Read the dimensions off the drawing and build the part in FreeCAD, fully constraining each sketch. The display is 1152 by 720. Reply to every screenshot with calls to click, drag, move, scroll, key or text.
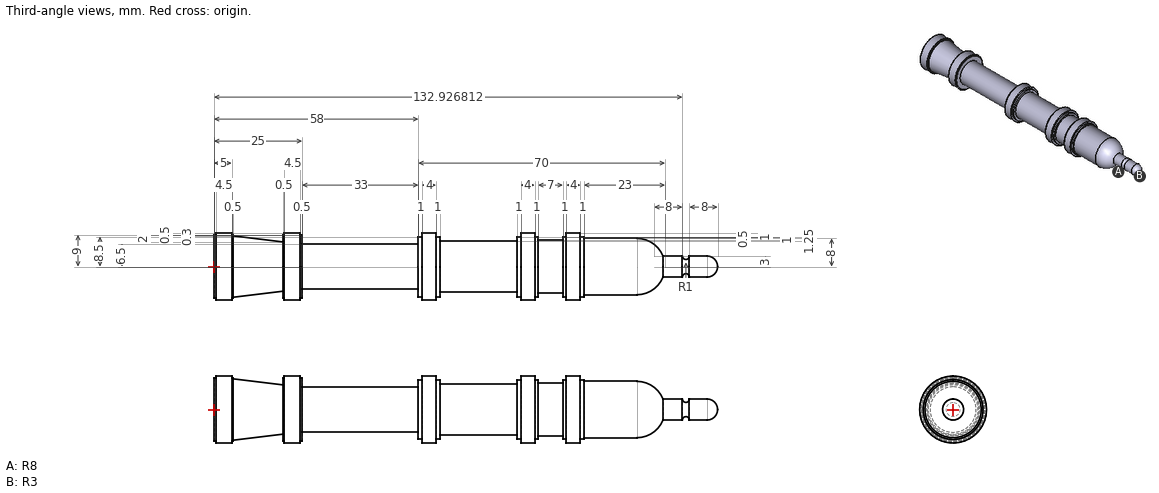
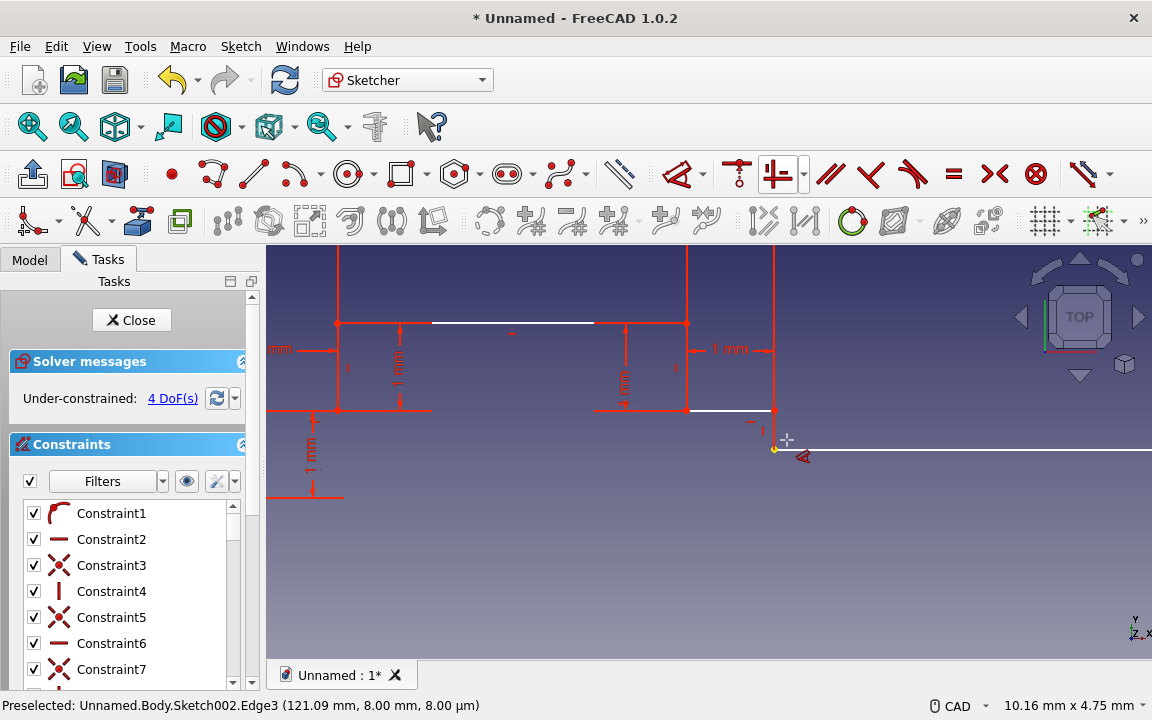
click(774, 430)
click(808, 430)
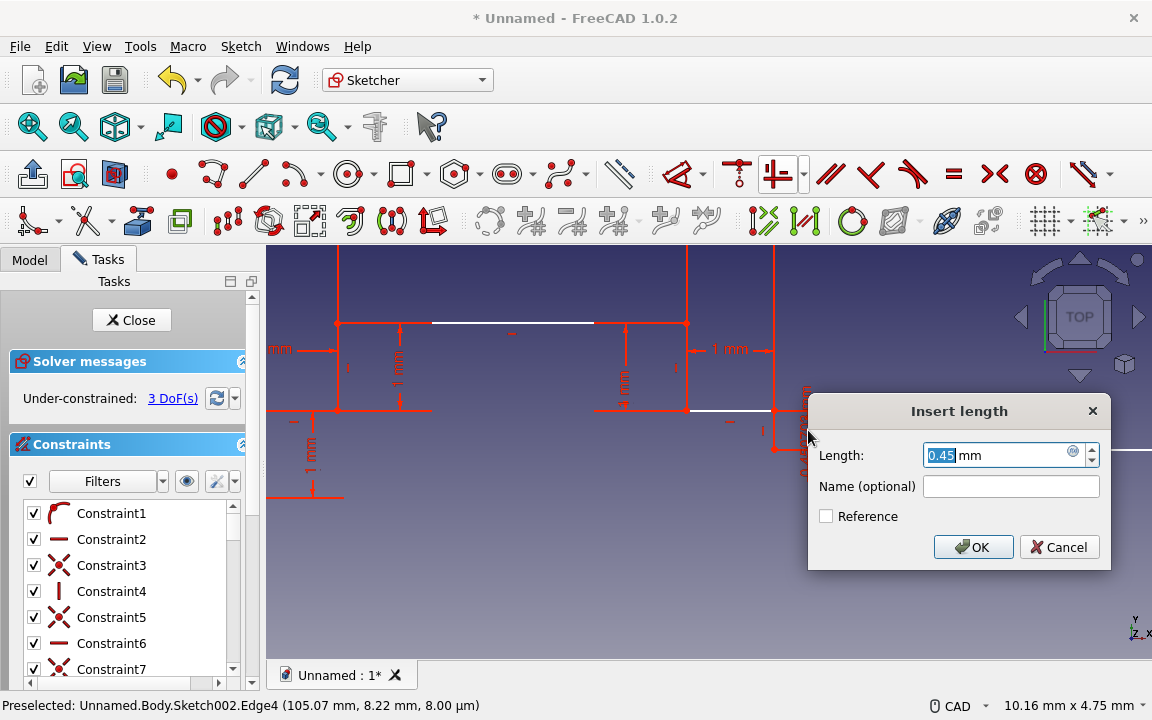
text(0.5)
key(Return)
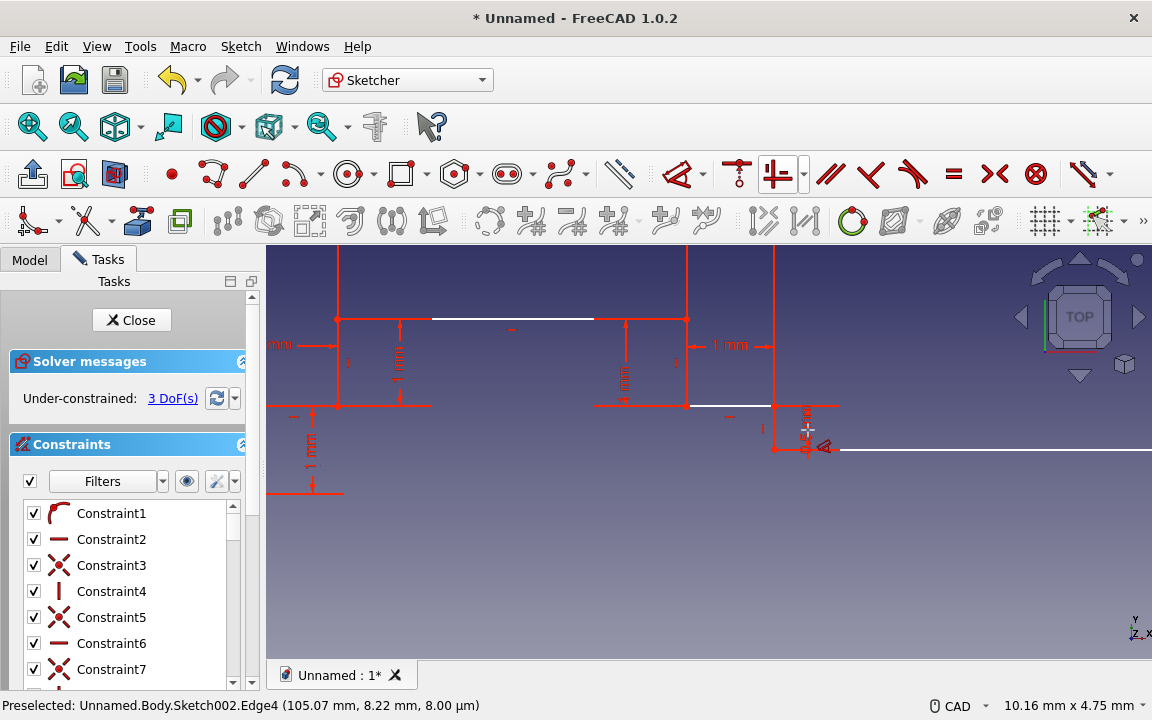
scroll(821, 437, down, 15)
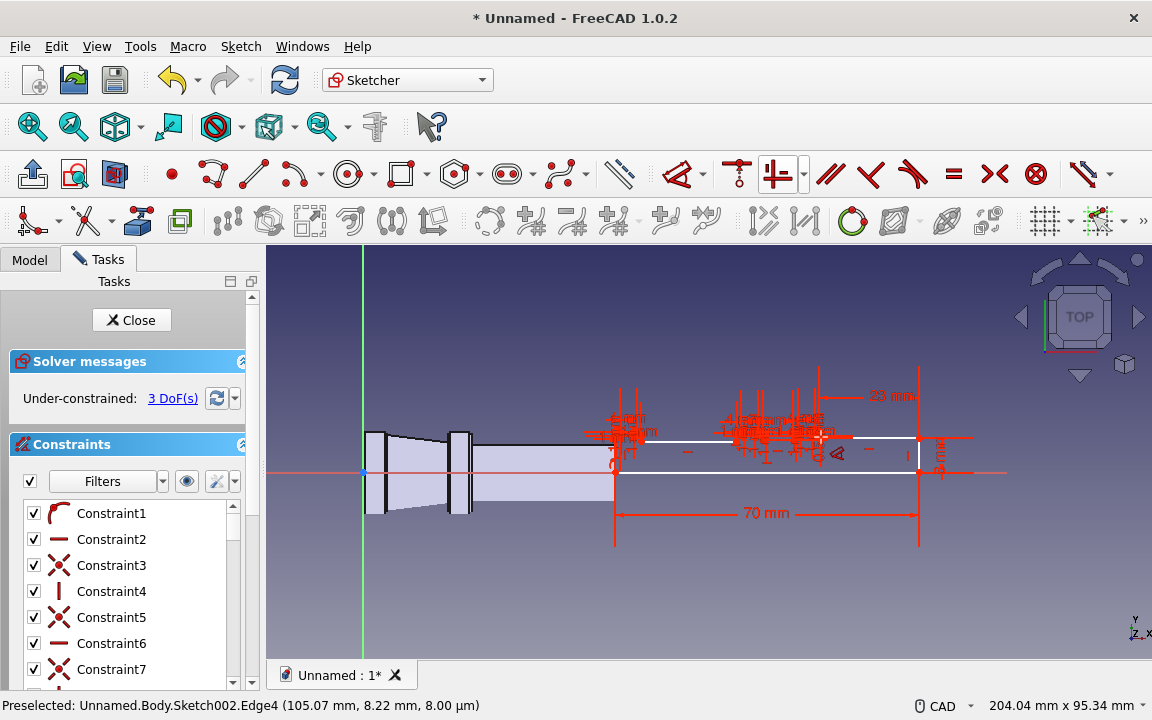
scroll(615, 447, up, 2)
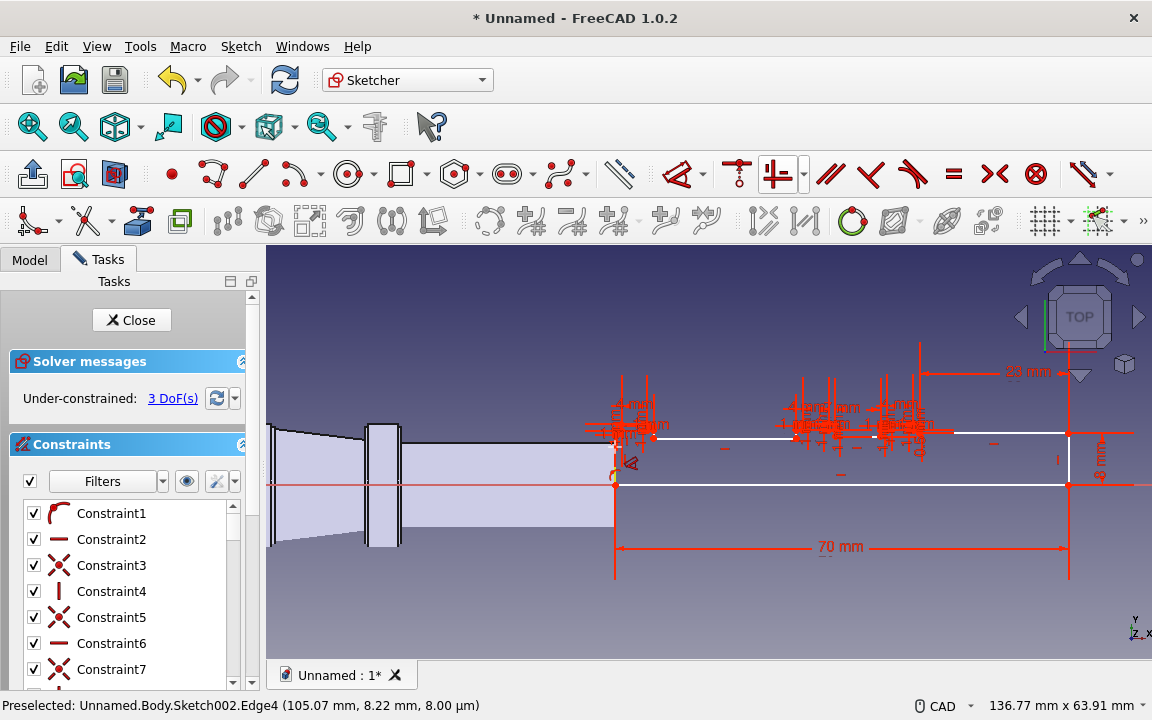
click(615, 447)
click(581, 458)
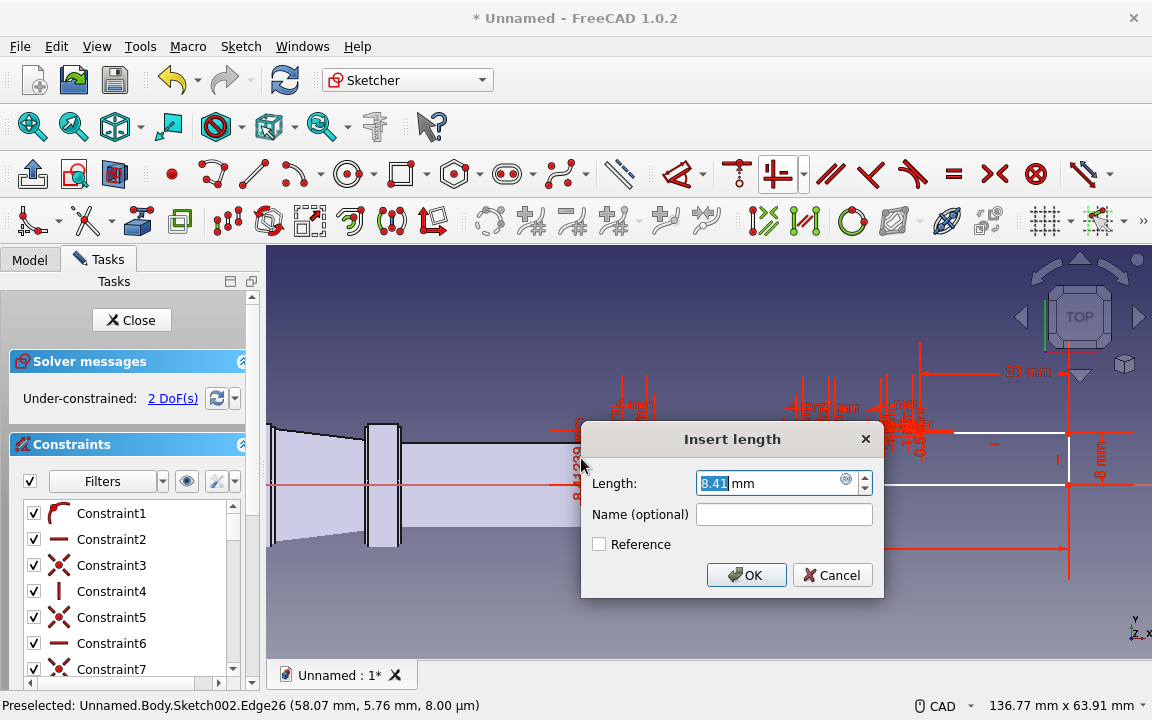
text(8.5)
key(Return)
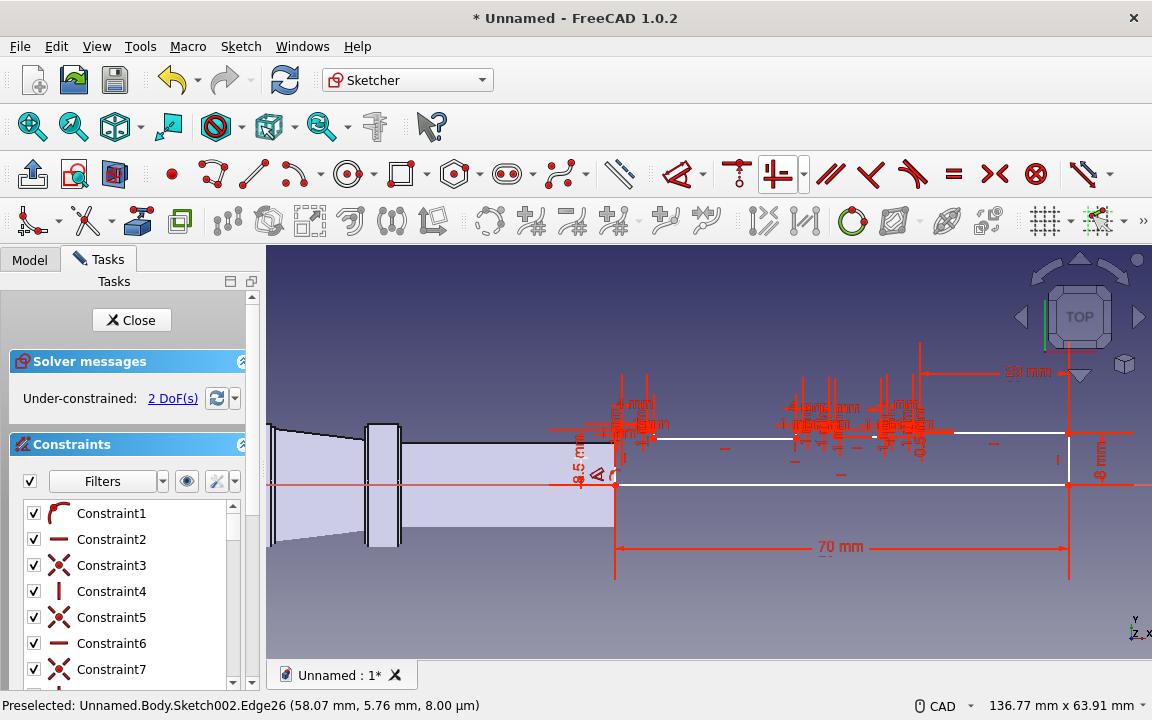
click(615, 485)
click(455, 519)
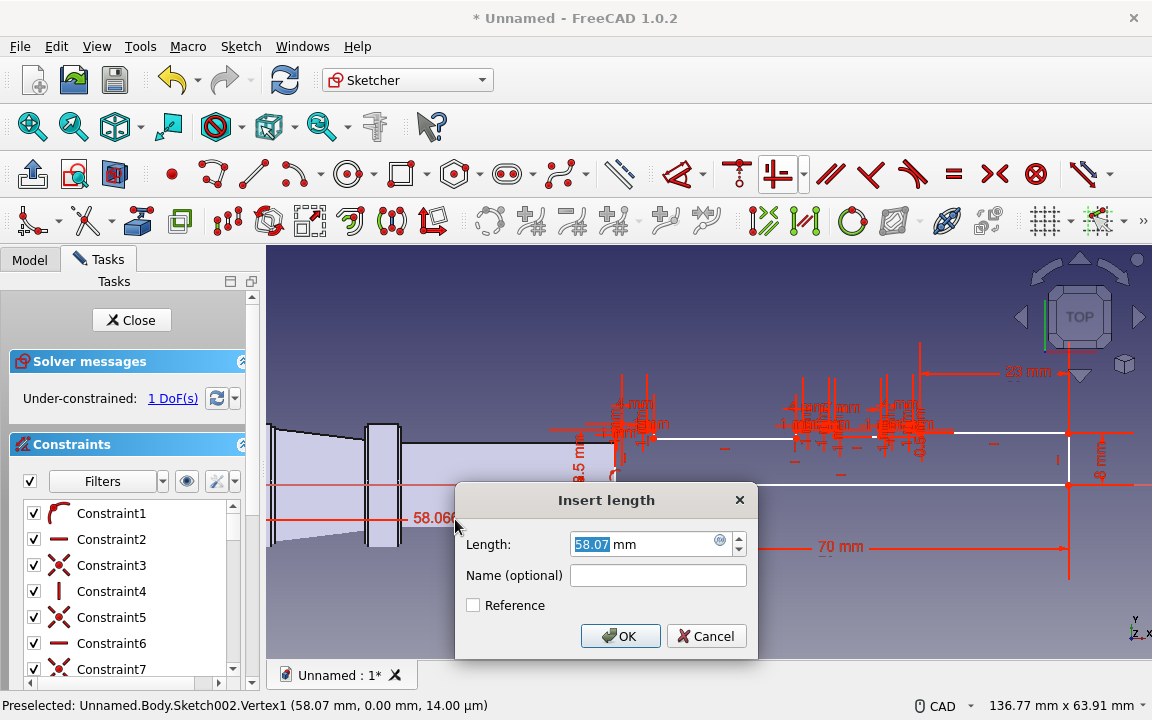
text(58)
key(Return)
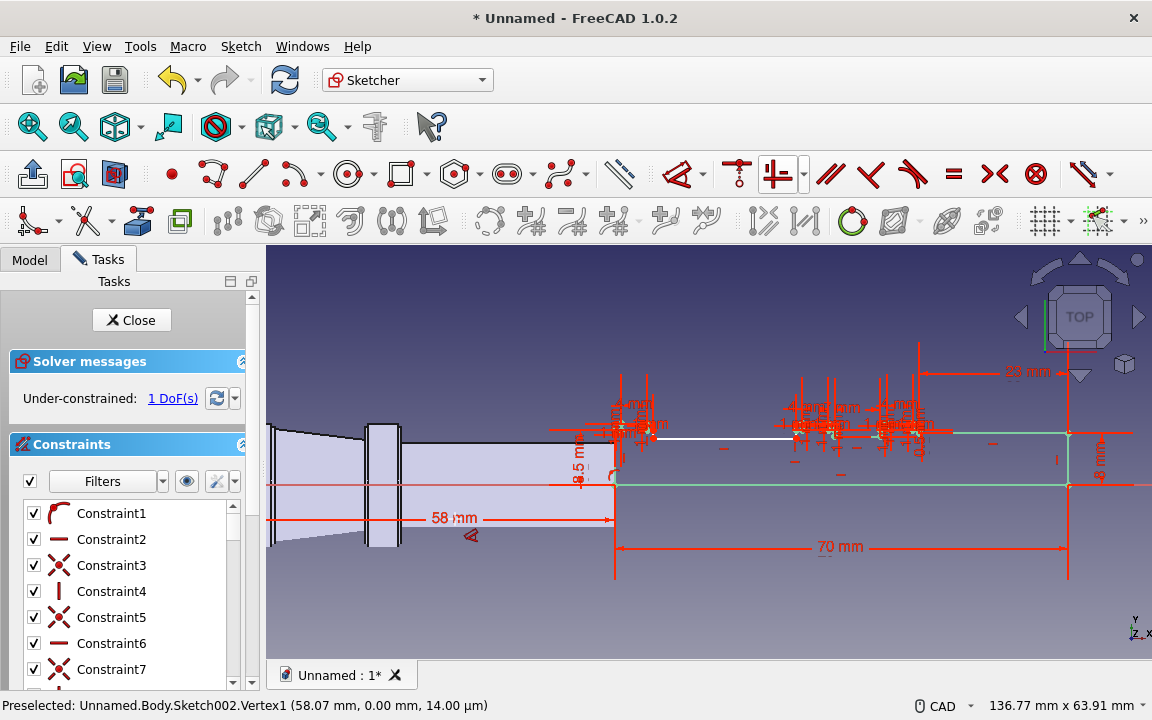
scroll(796, 434, up, 8)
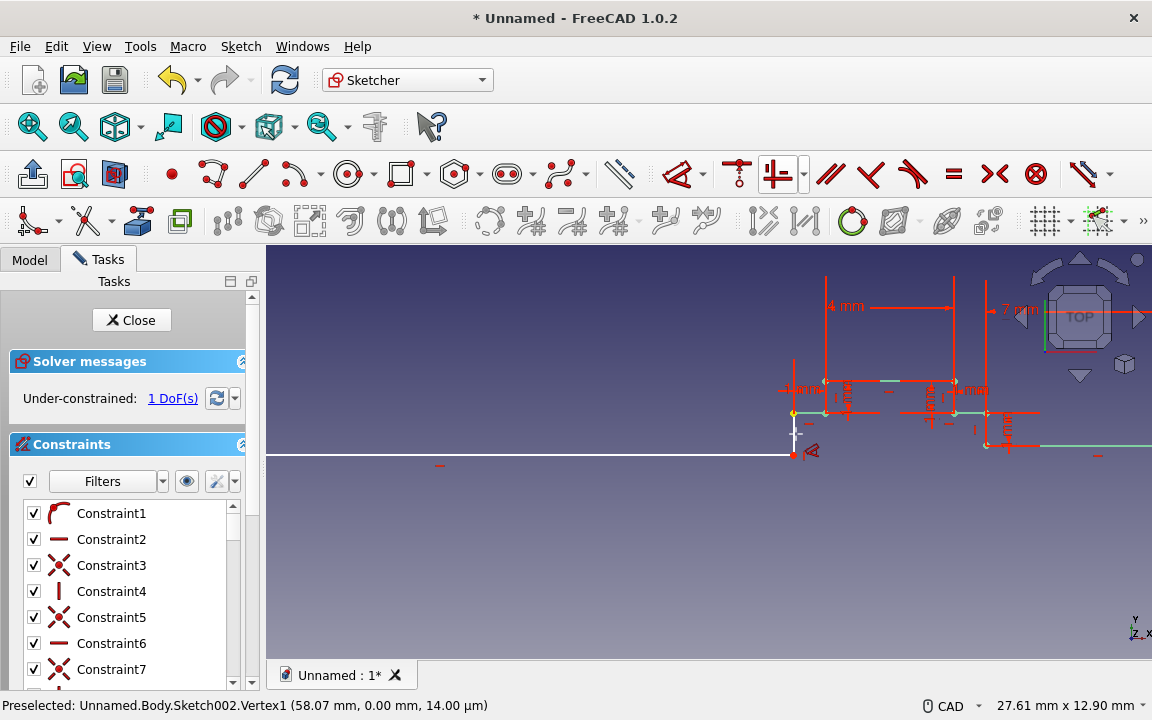
click(794, 434)
click(828, 434)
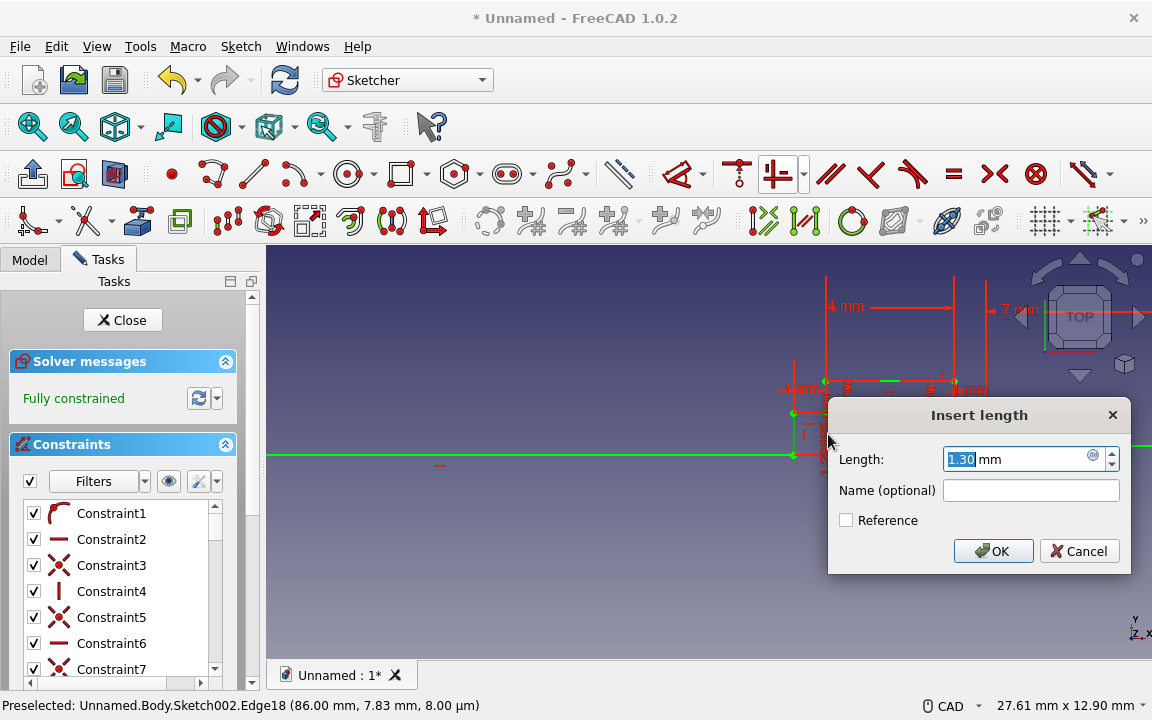
text(1.25)
key(Return)
key(Escape)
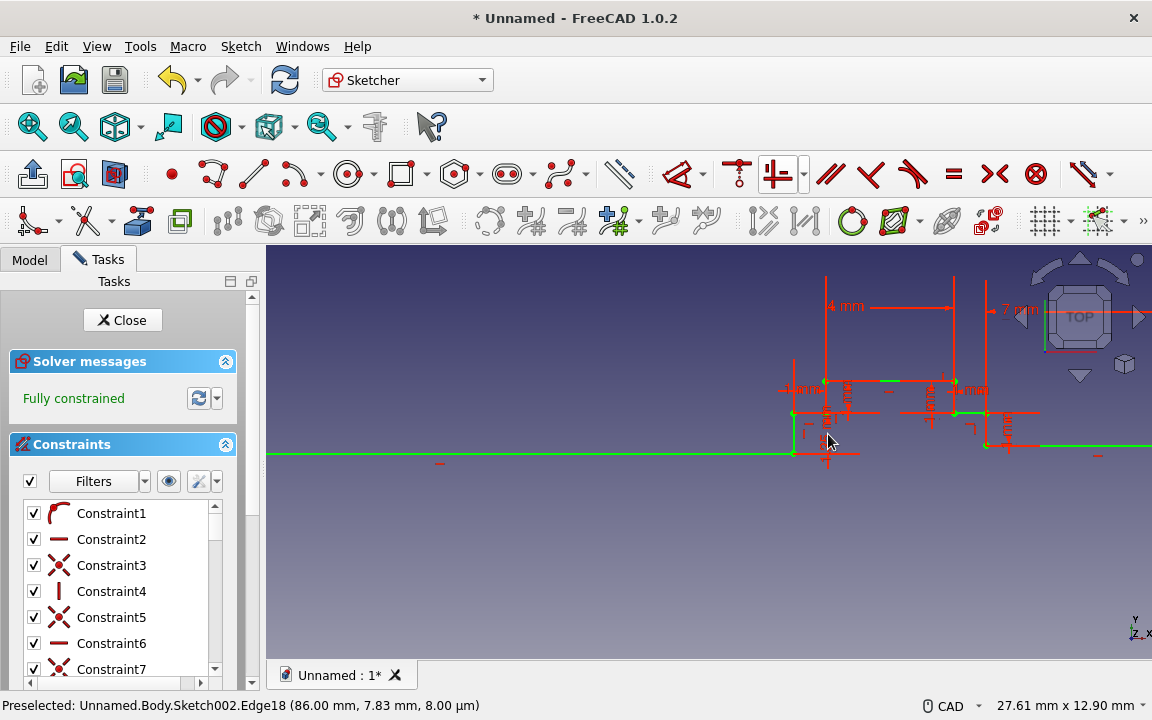
click(123, 320)